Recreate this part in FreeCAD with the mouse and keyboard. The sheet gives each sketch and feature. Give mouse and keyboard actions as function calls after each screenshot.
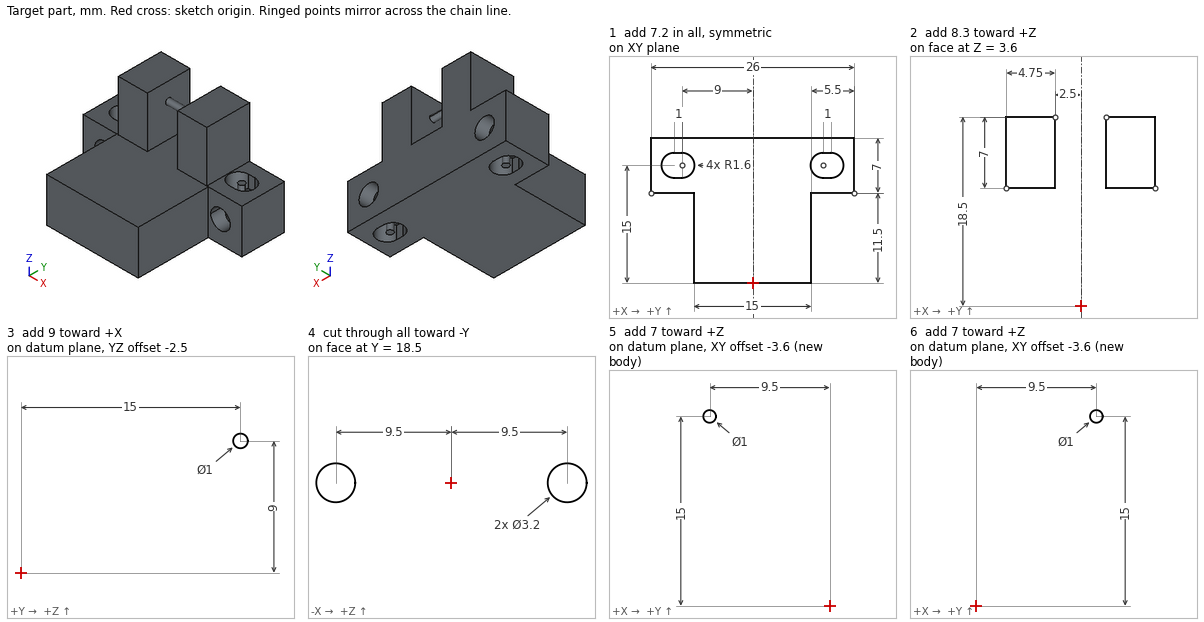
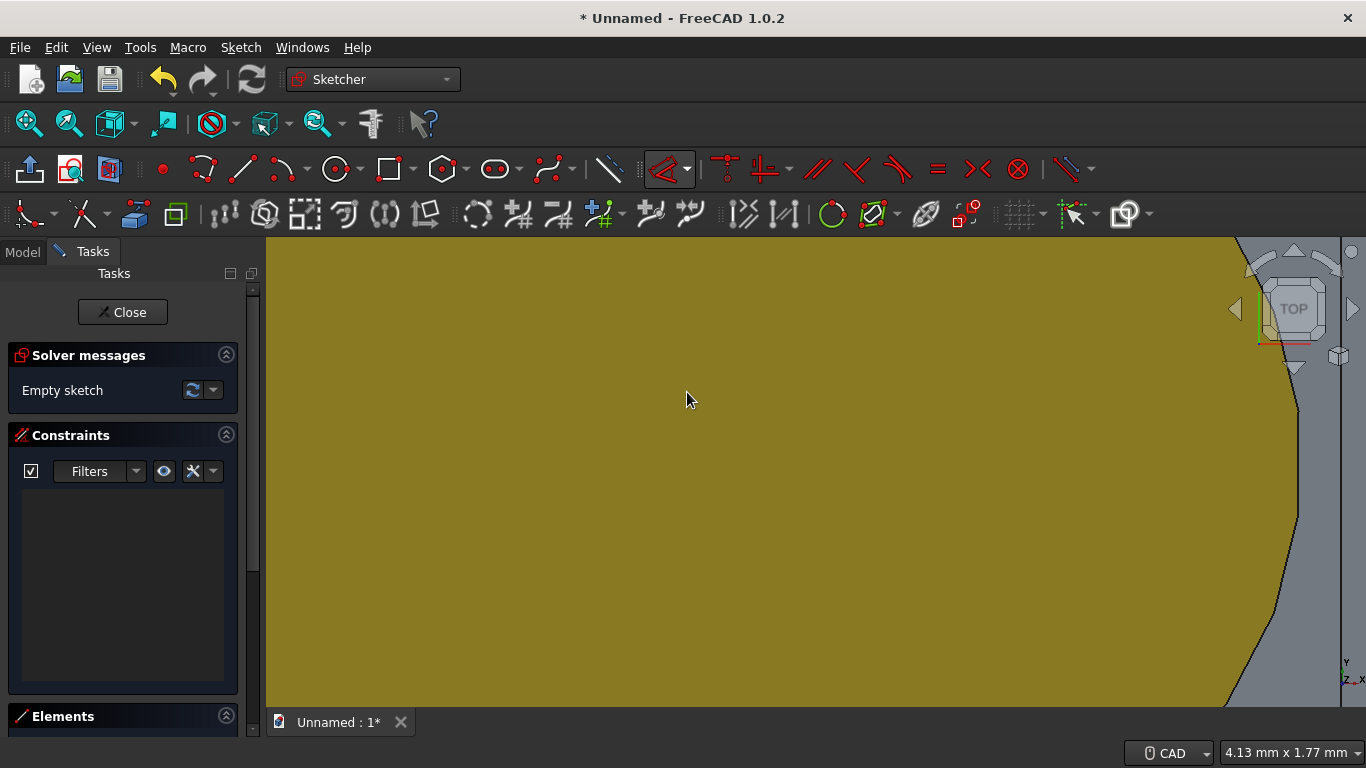
key(g)
key(c)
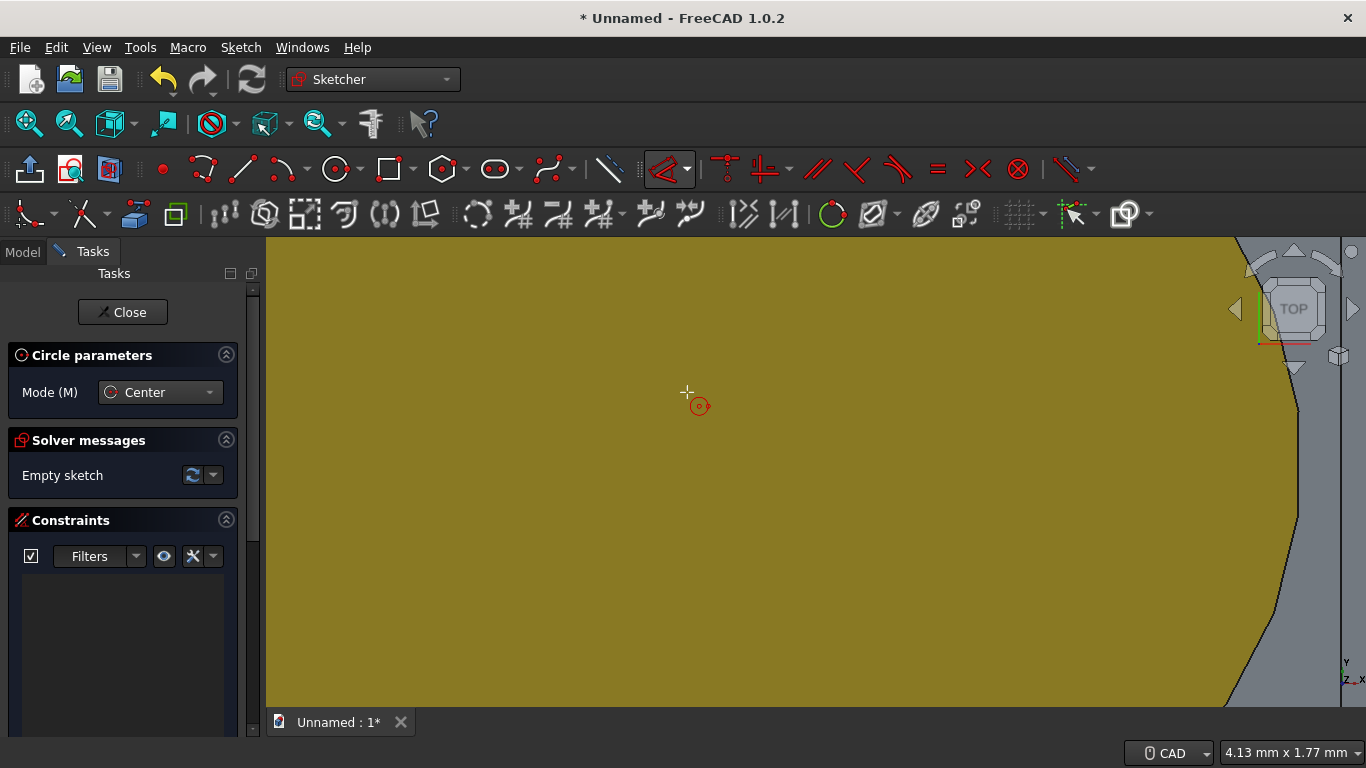
click(743, 462)
click(837, 368)
key(Escape)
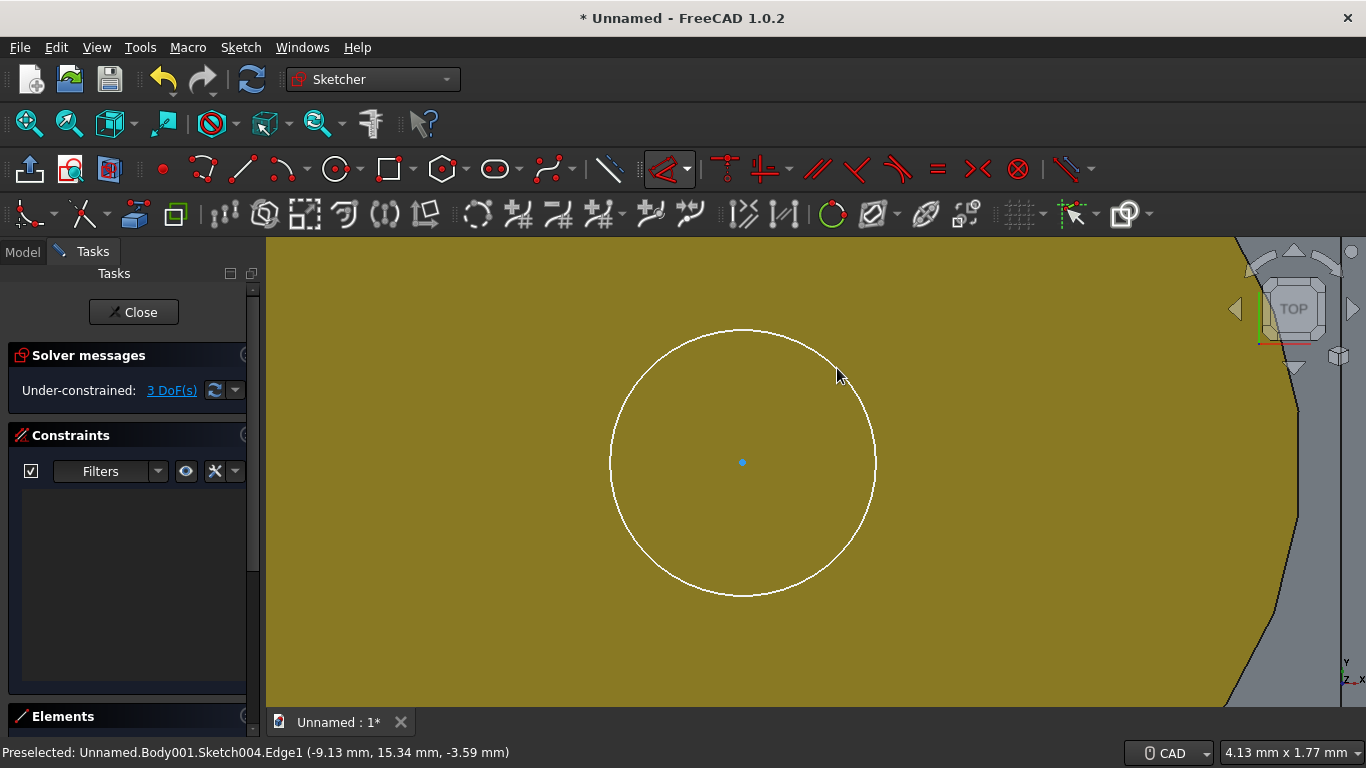
click(837, 369)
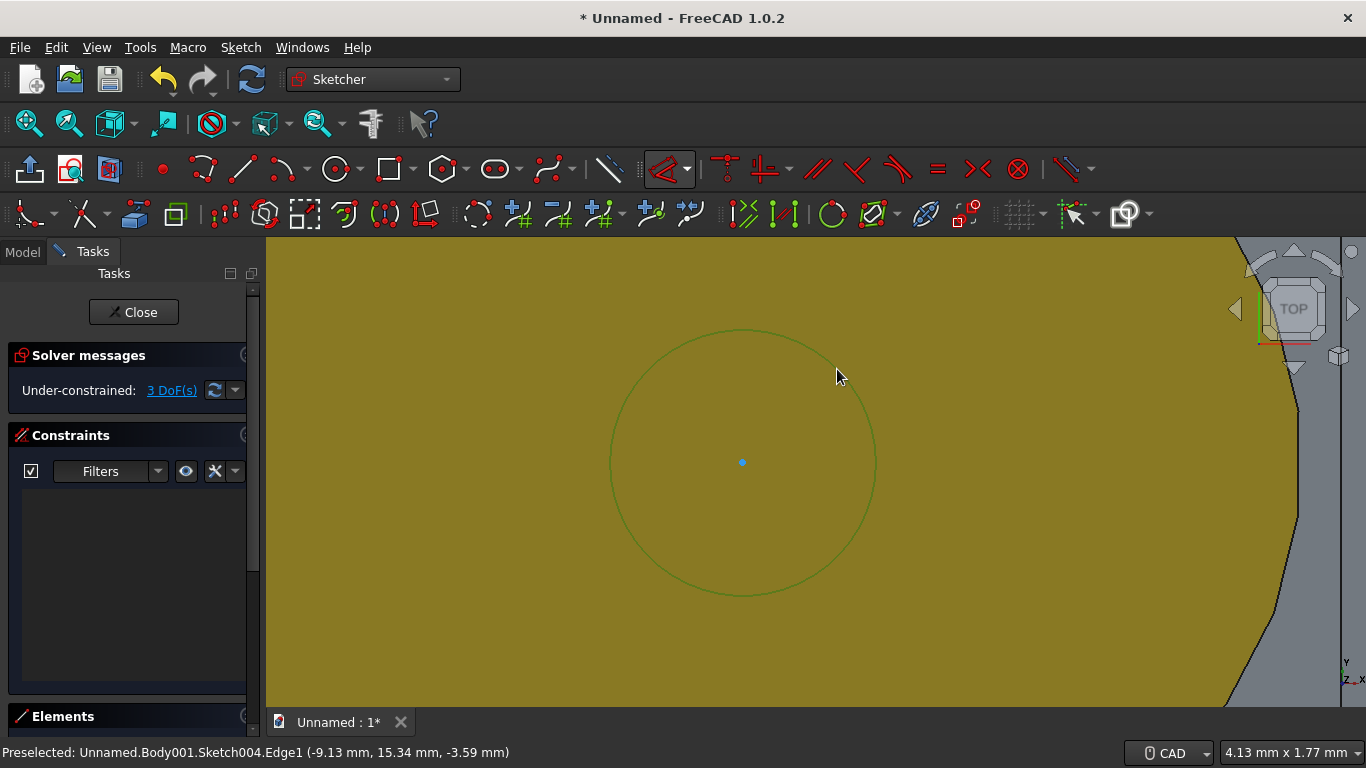
key(k)
key(o)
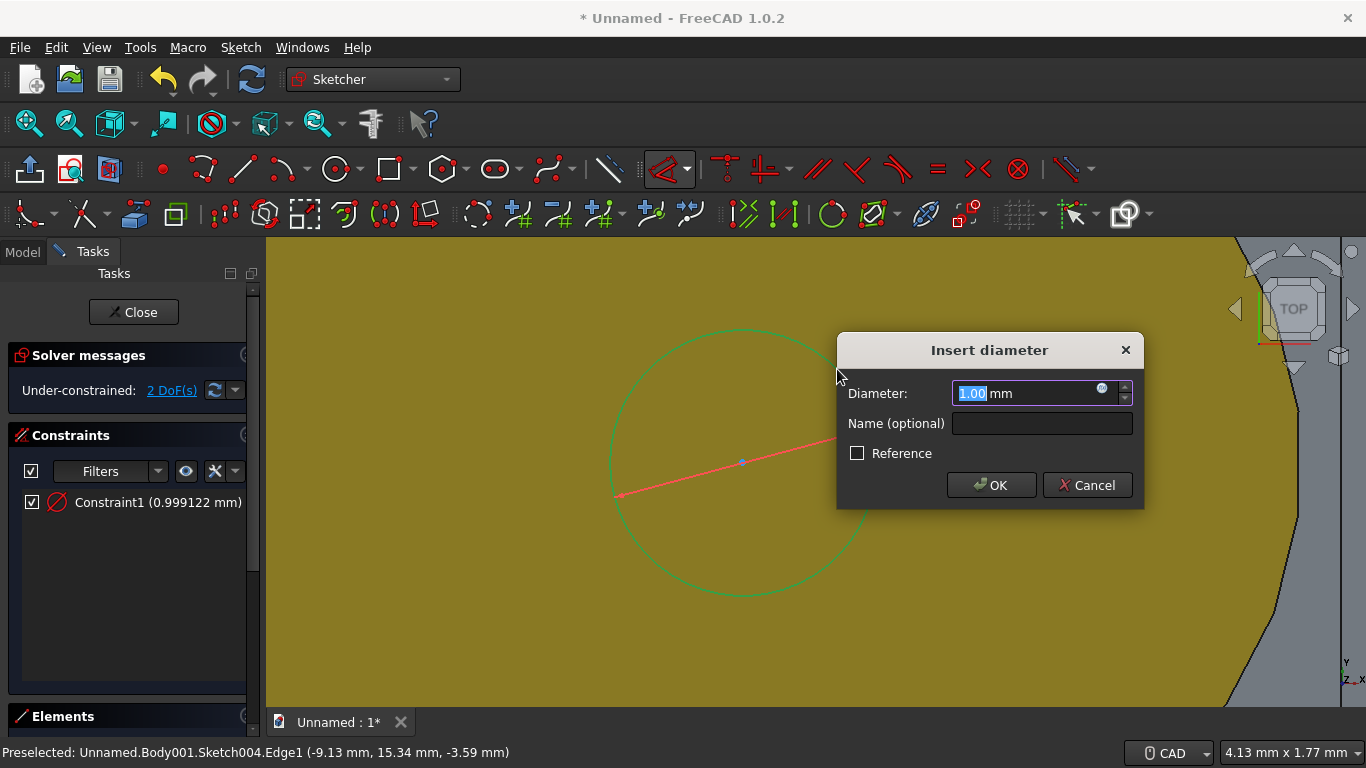
text(1)
key(Return)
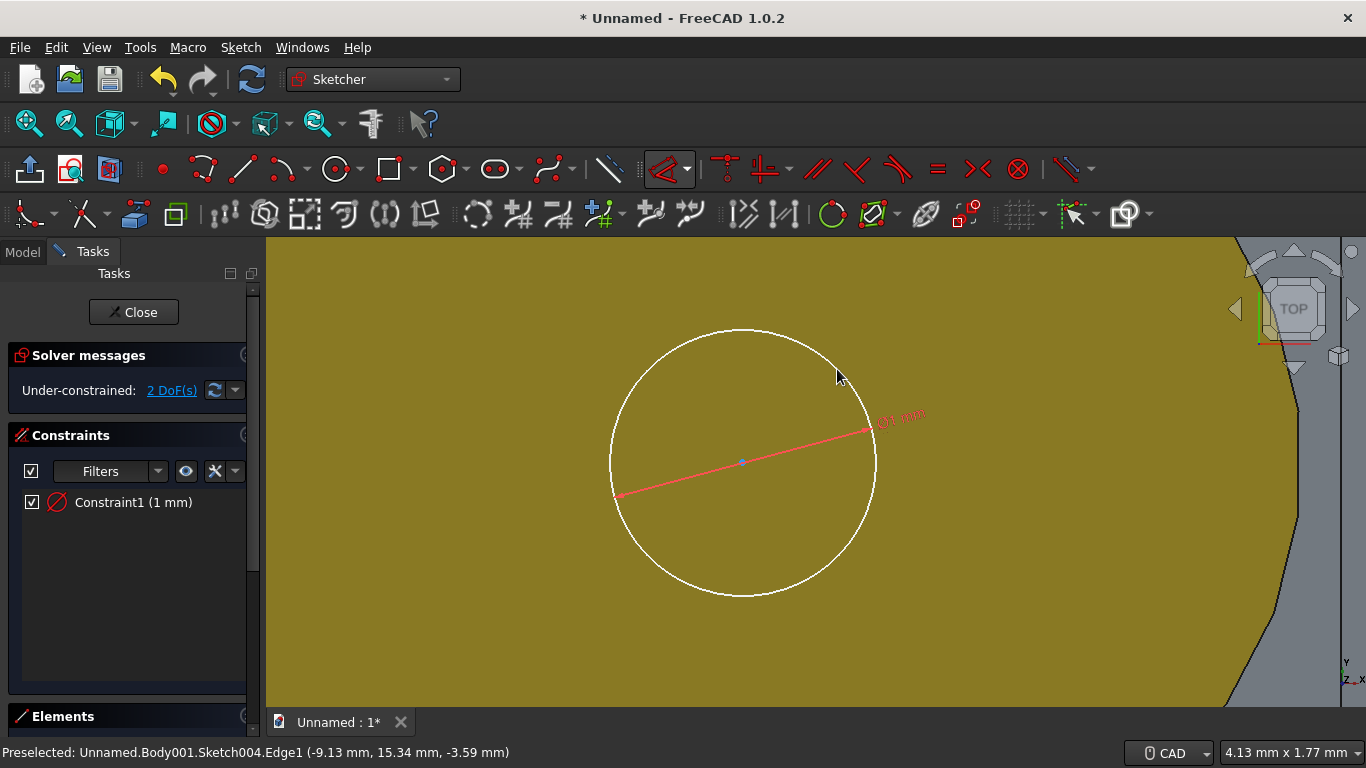
click(743, 463)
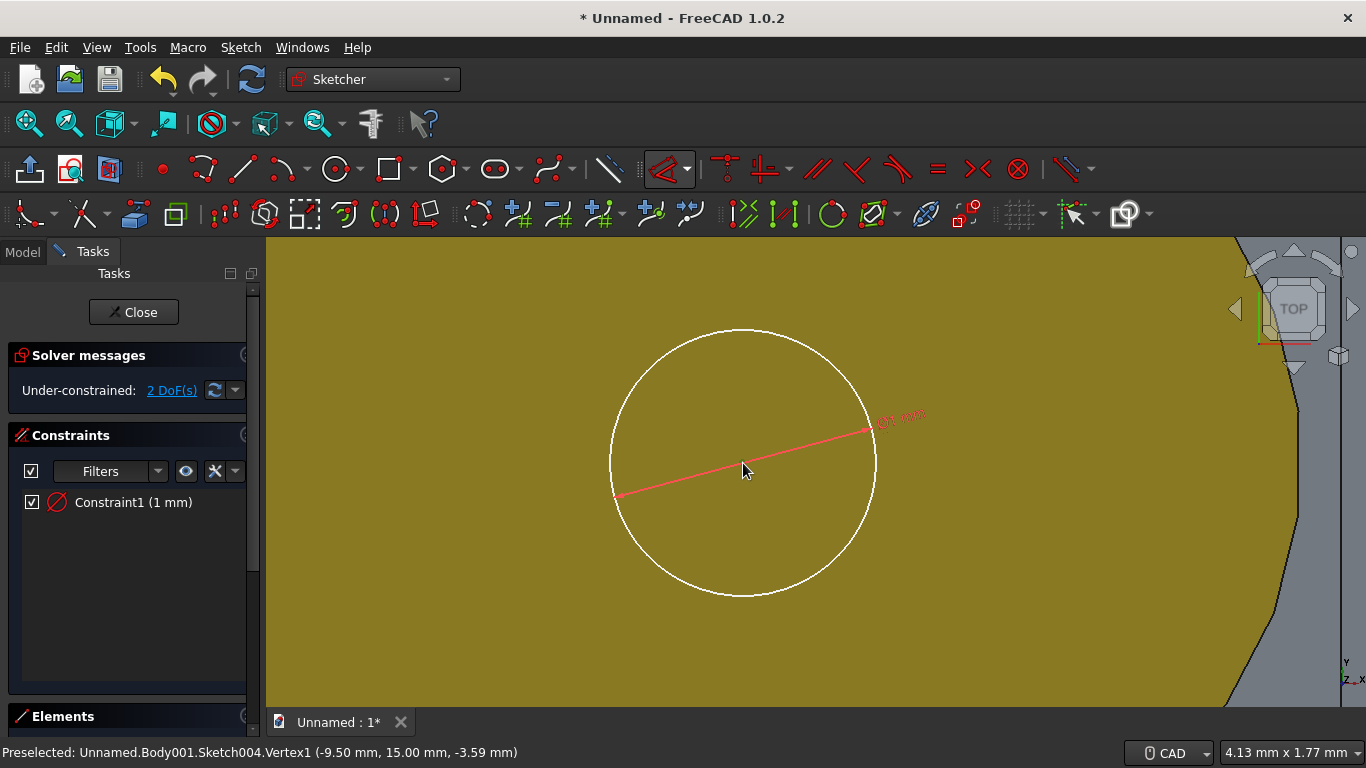
key(i)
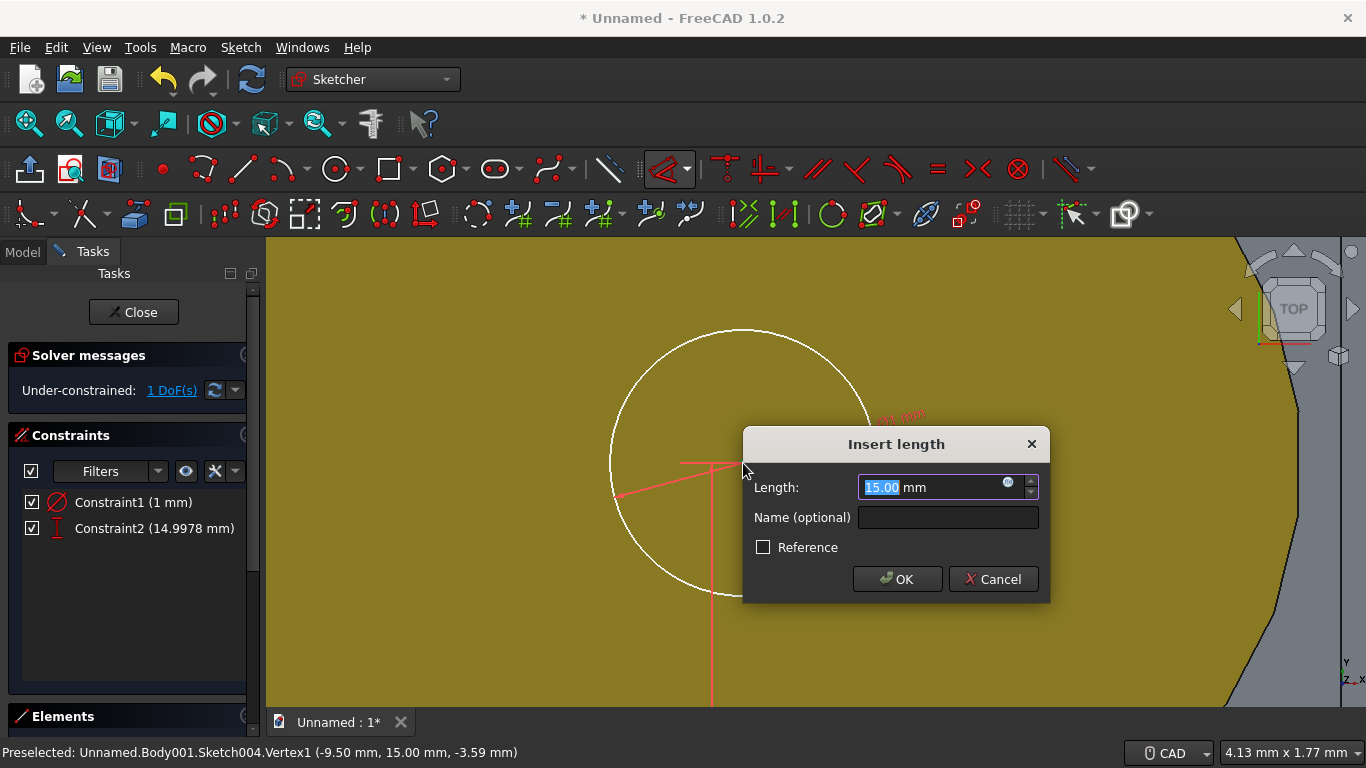
text(15)
key(Return)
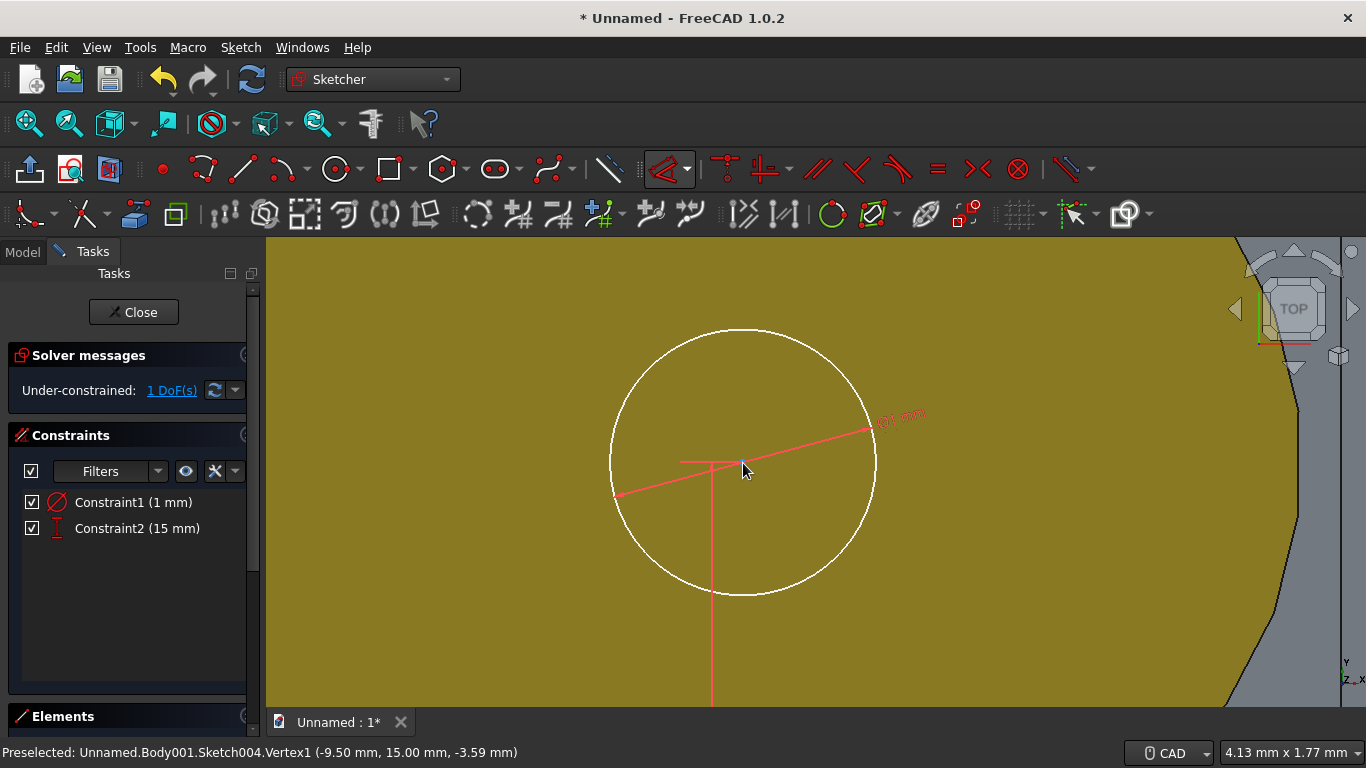
click(743, 462)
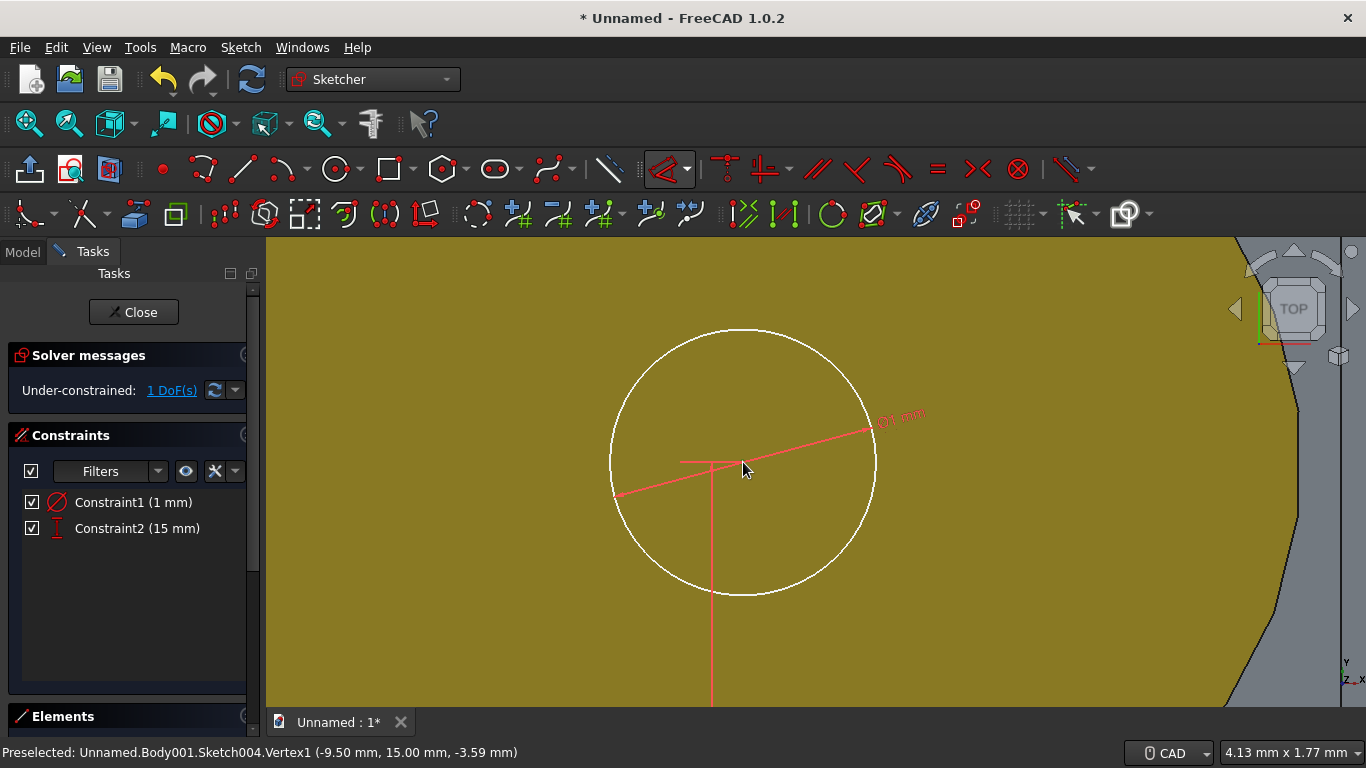
key(l)